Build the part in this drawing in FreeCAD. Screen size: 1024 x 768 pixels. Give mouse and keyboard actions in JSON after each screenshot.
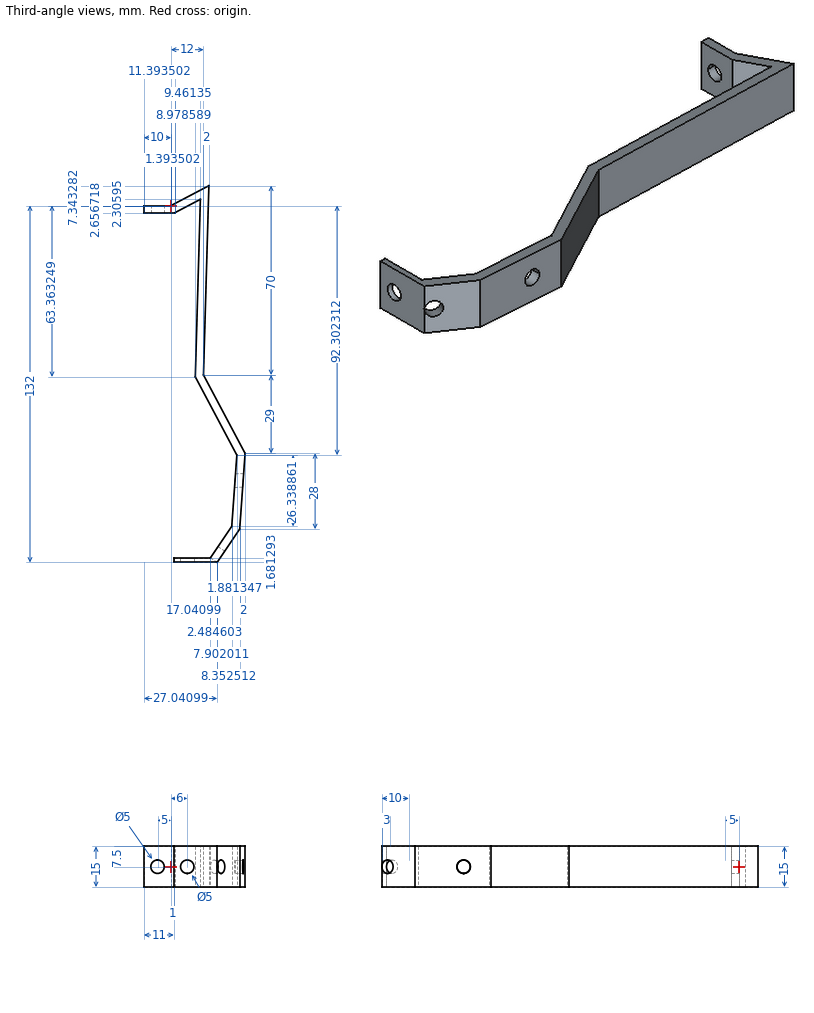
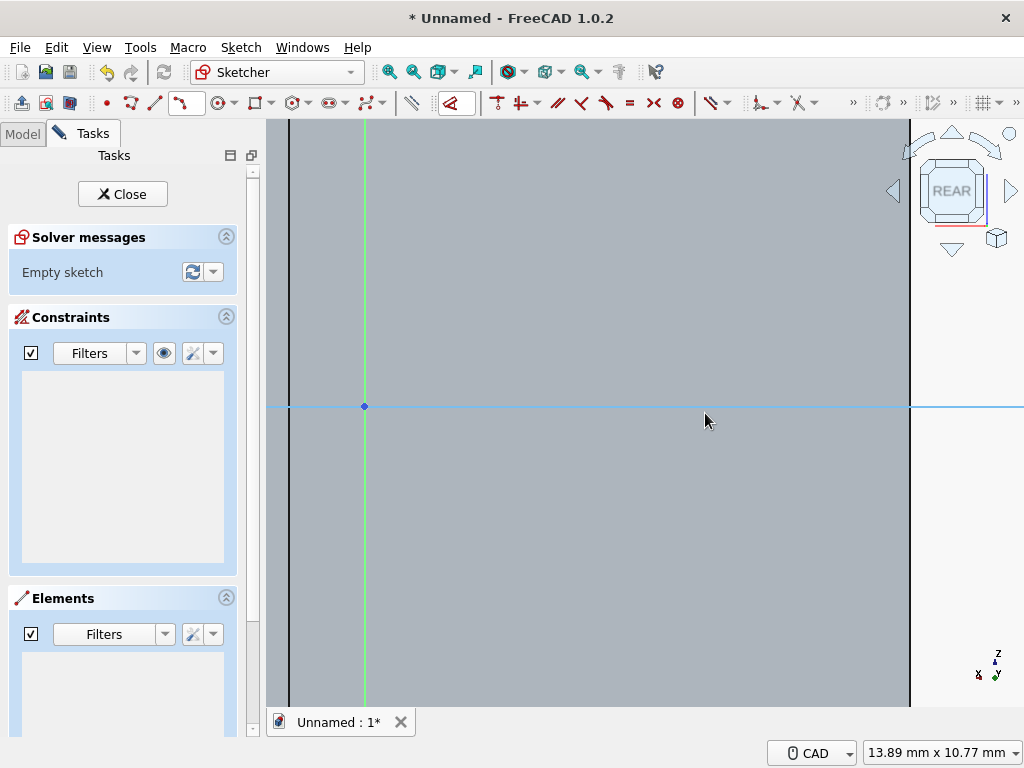
{"action": "left_click", "coordinate": [218, 104]}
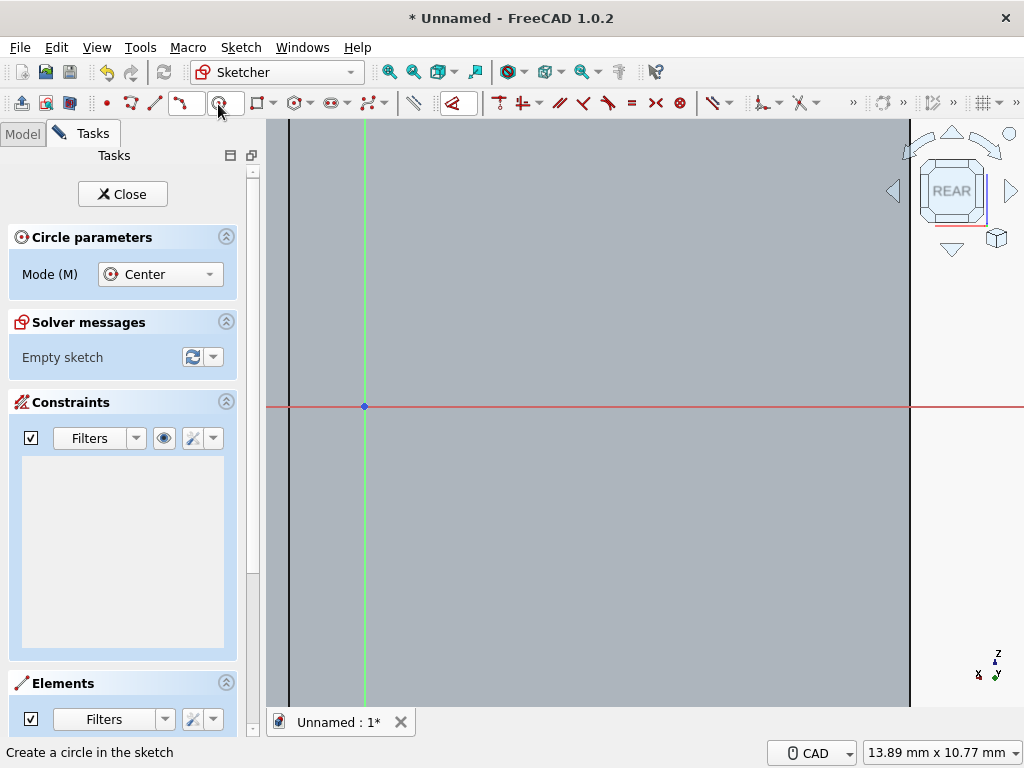
{"action": "left_click", "coordinate": [637, 407]}
{"action": "mouse_move", "coordinate": [734, 310]}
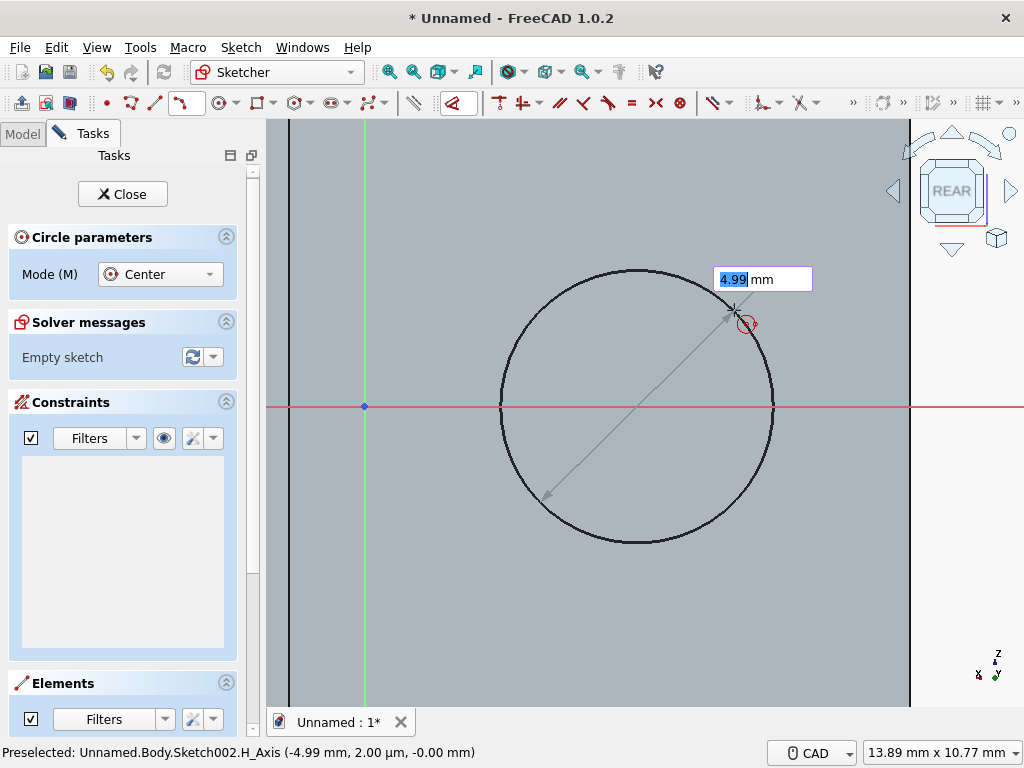
{"action": "type", "text": "5"}
{"action": "key", "text": "Return"}
{"action": "key", "text": "Escape"}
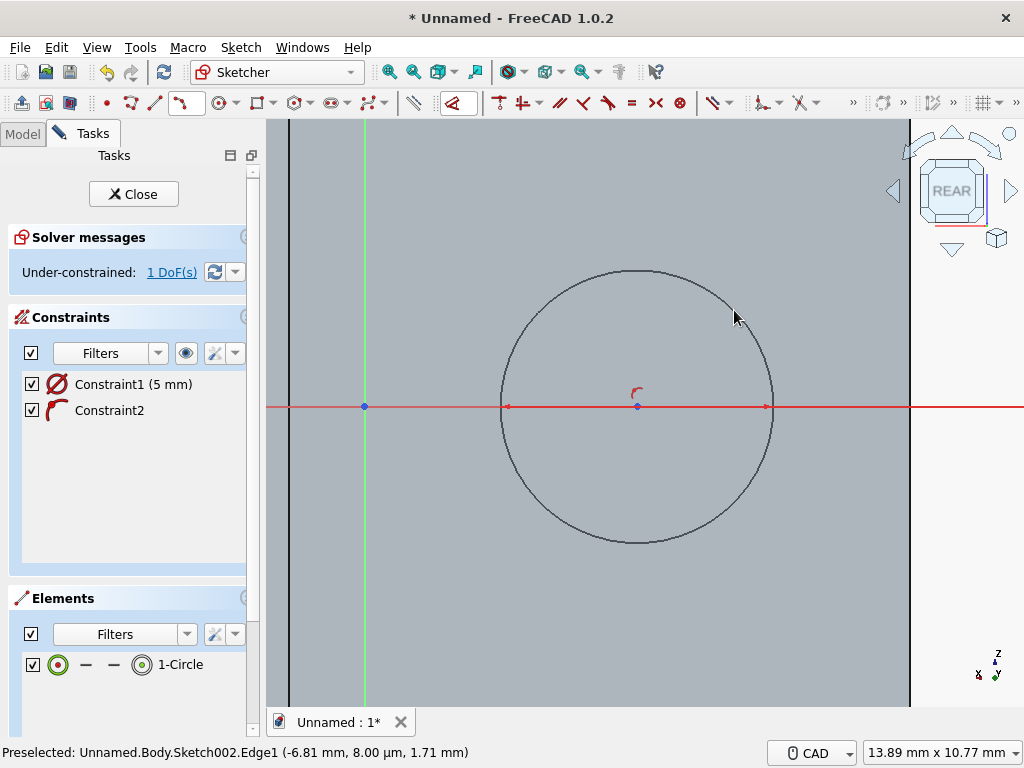
{"action": "left_click", "coordinate": [637, 407]}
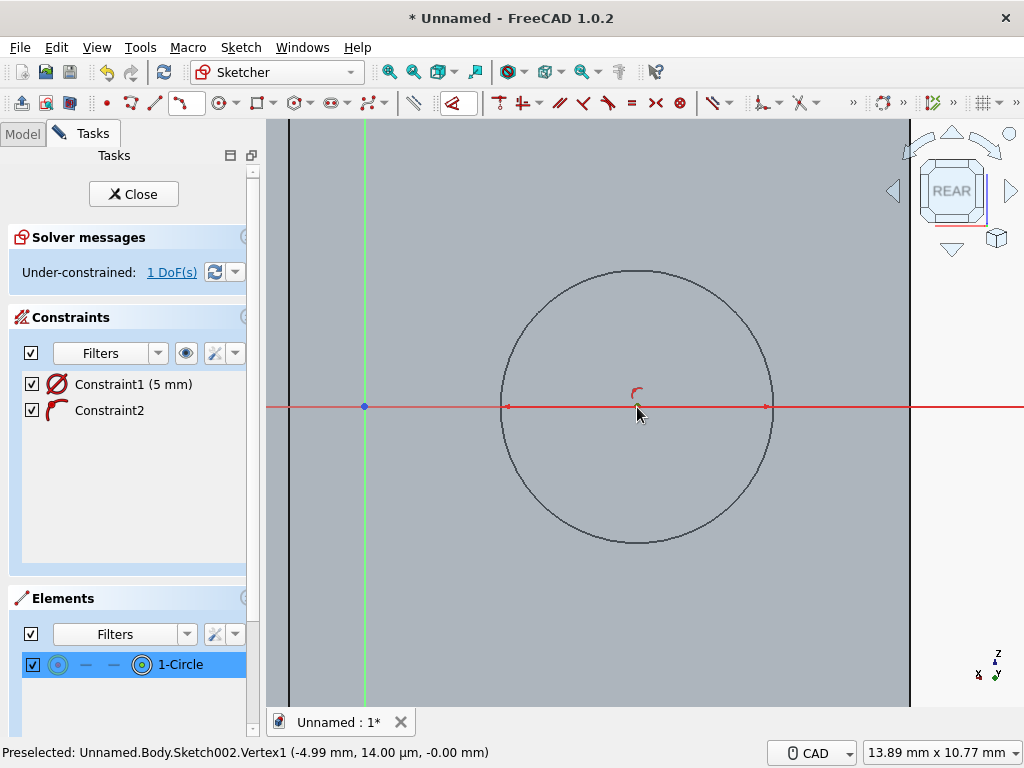
{"action": "left_click", "coordinate": [472, 104]}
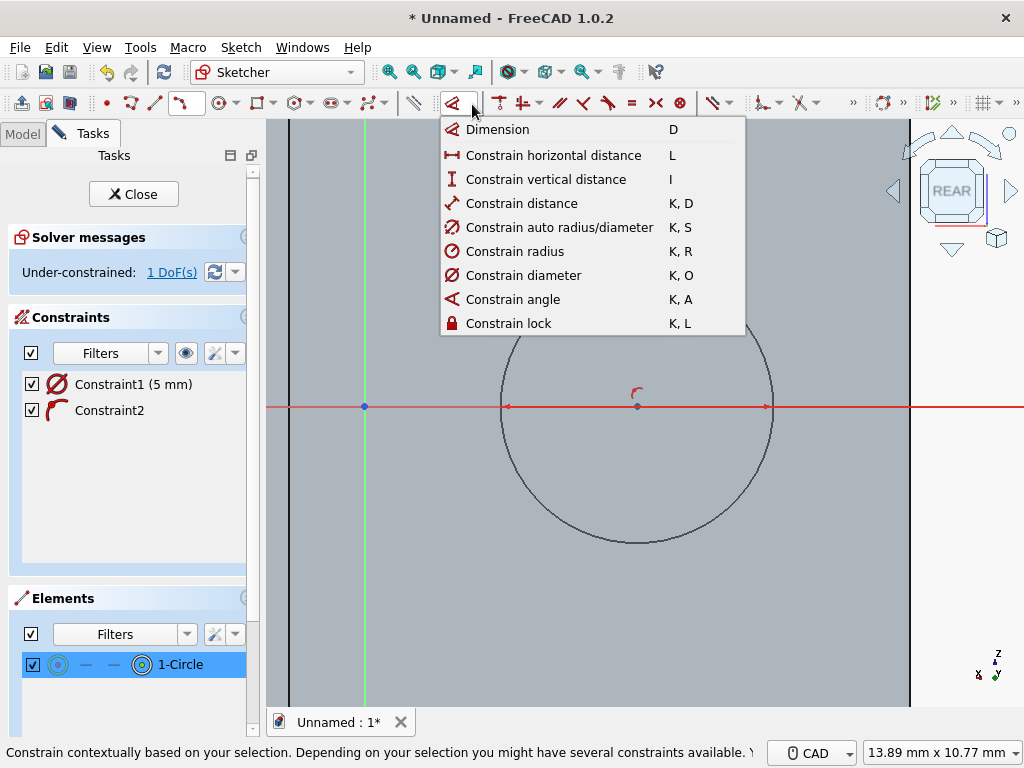
{"action": "left_click", "coordinate": [593, 155]}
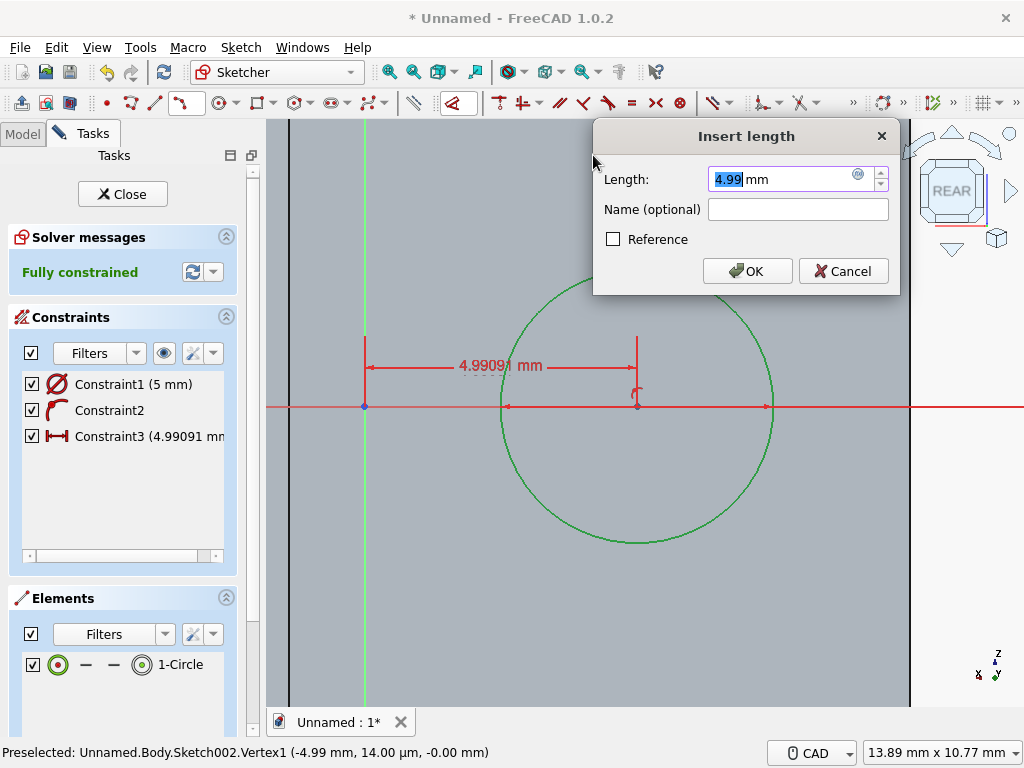
{"action": "type", "text": "5"}
{"action": "key", "text": "Return"}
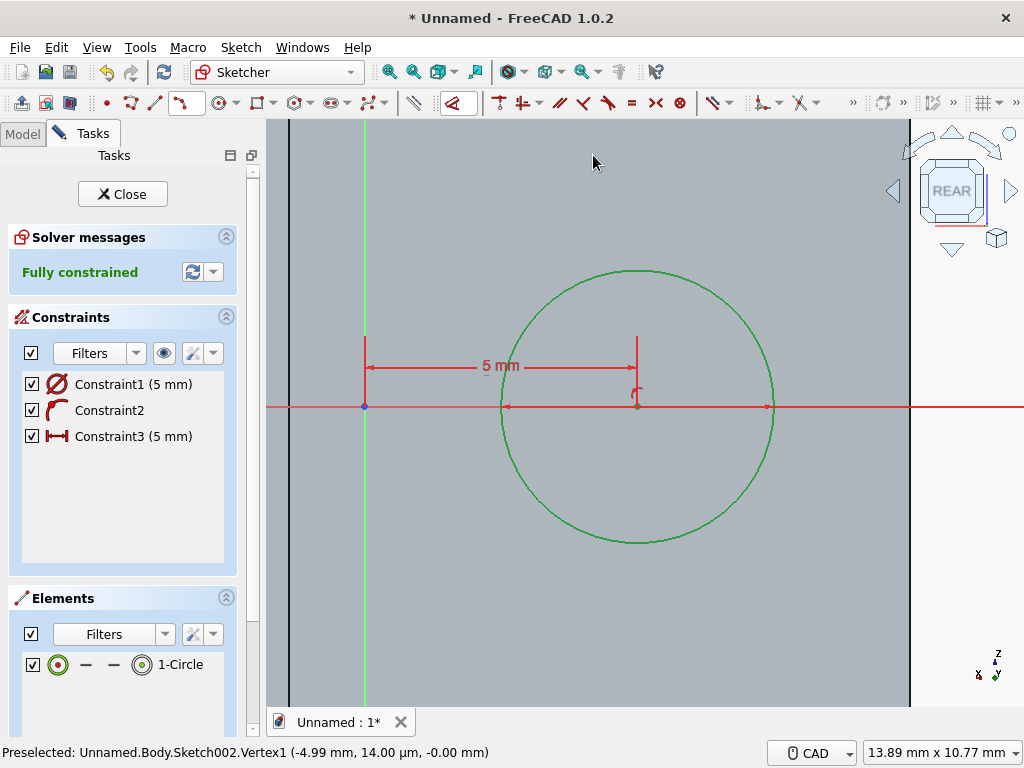
{"action": "left_click", "coordinate": [123, 194]}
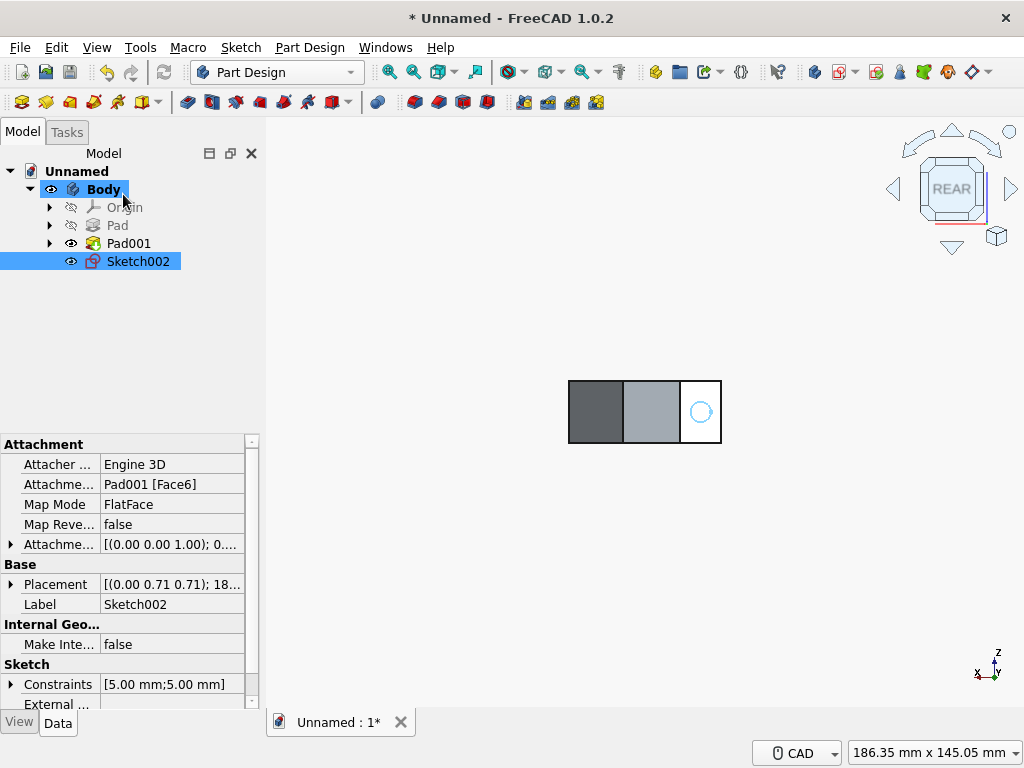
{"action": "left_click", "coordinate": [188, 102]}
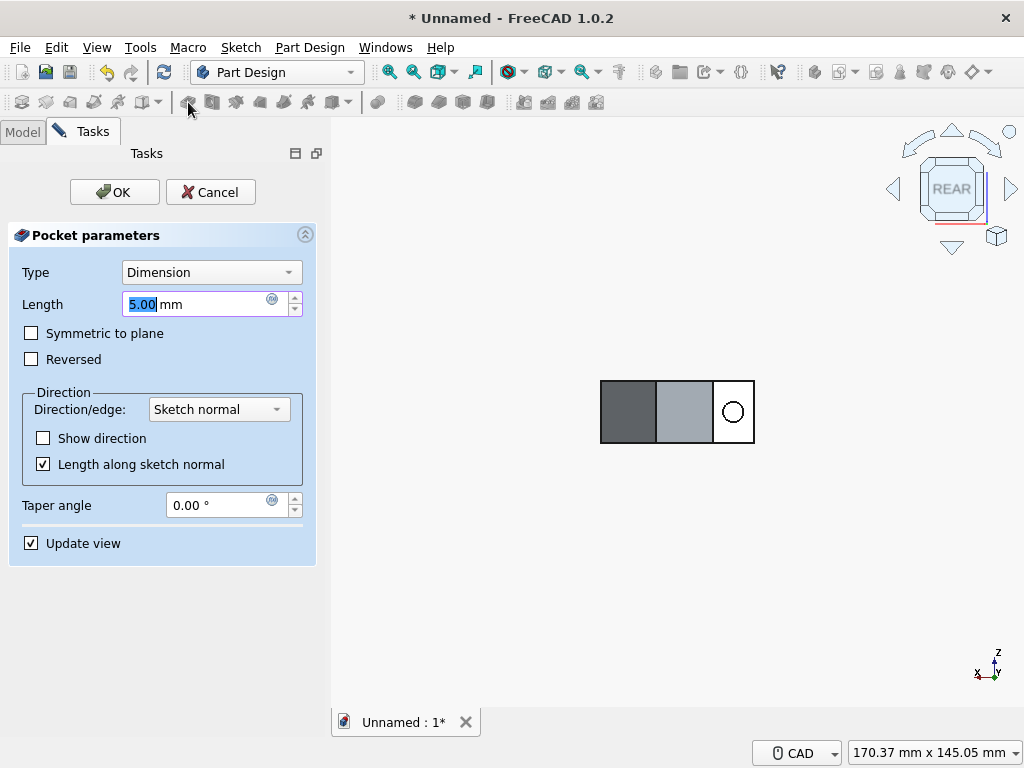
{"action": "type", "text": "5"}
{"action": "key", "text": "Tab"}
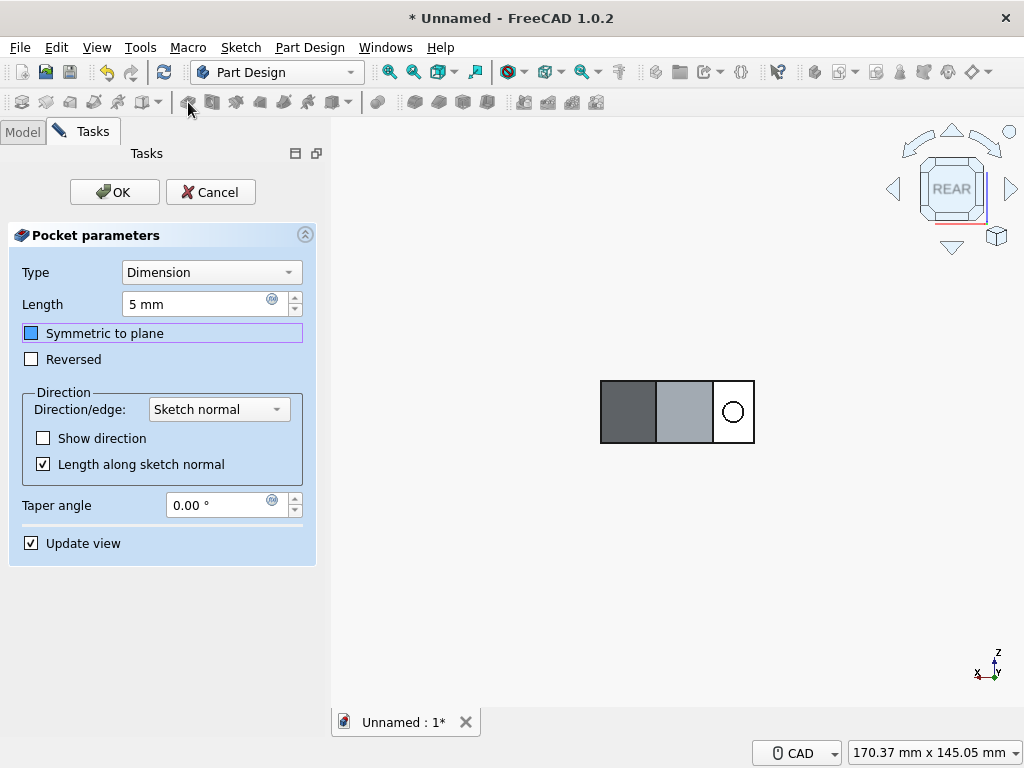
{"action": "left_click", "coordinate": [115, 192]}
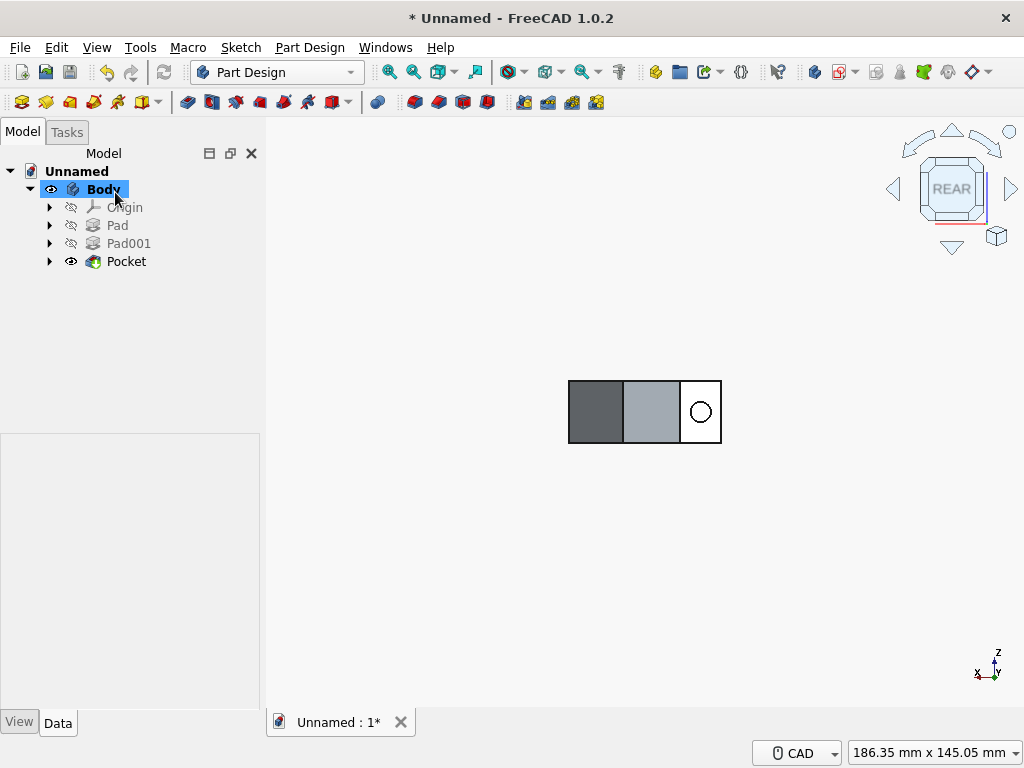
{"action": "left_click", "coordinate": [390, 72]}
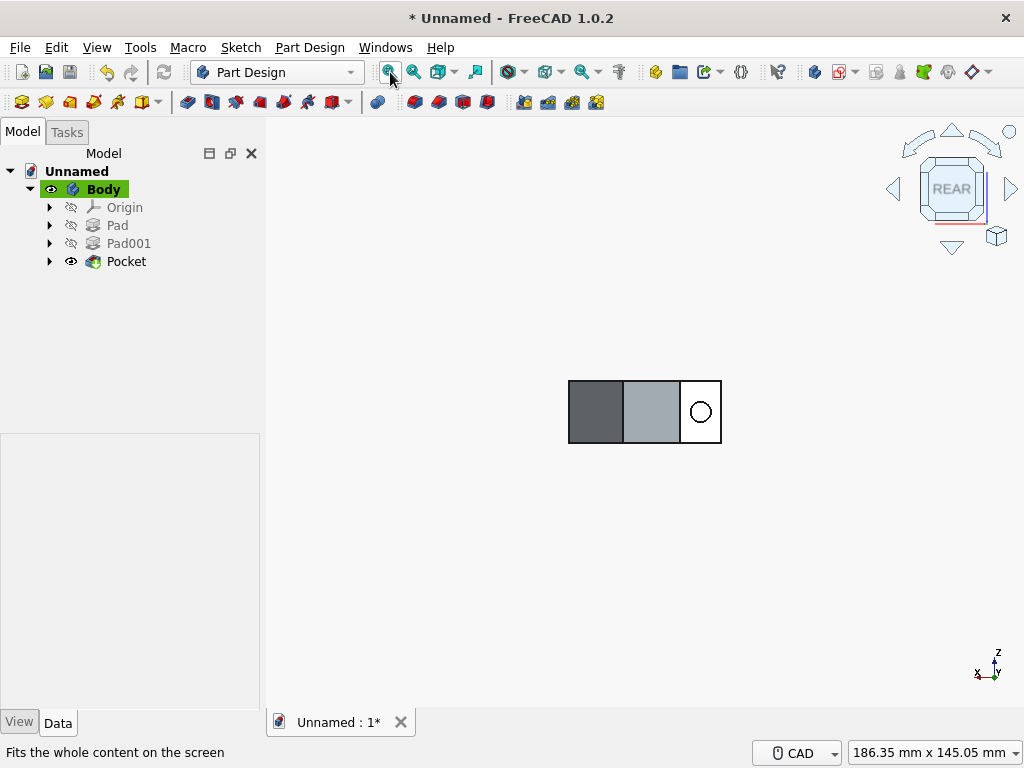
{"action": "key", "text": "0"}